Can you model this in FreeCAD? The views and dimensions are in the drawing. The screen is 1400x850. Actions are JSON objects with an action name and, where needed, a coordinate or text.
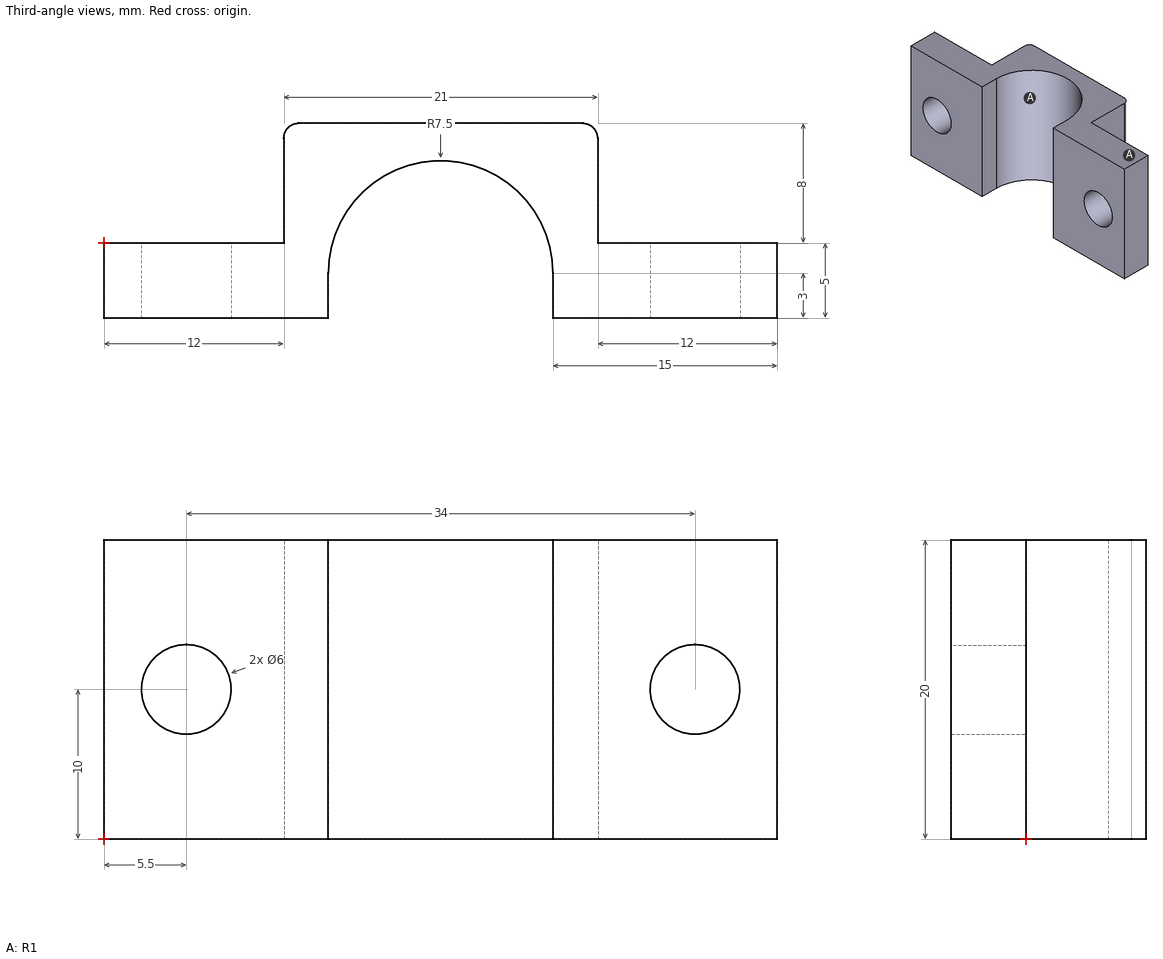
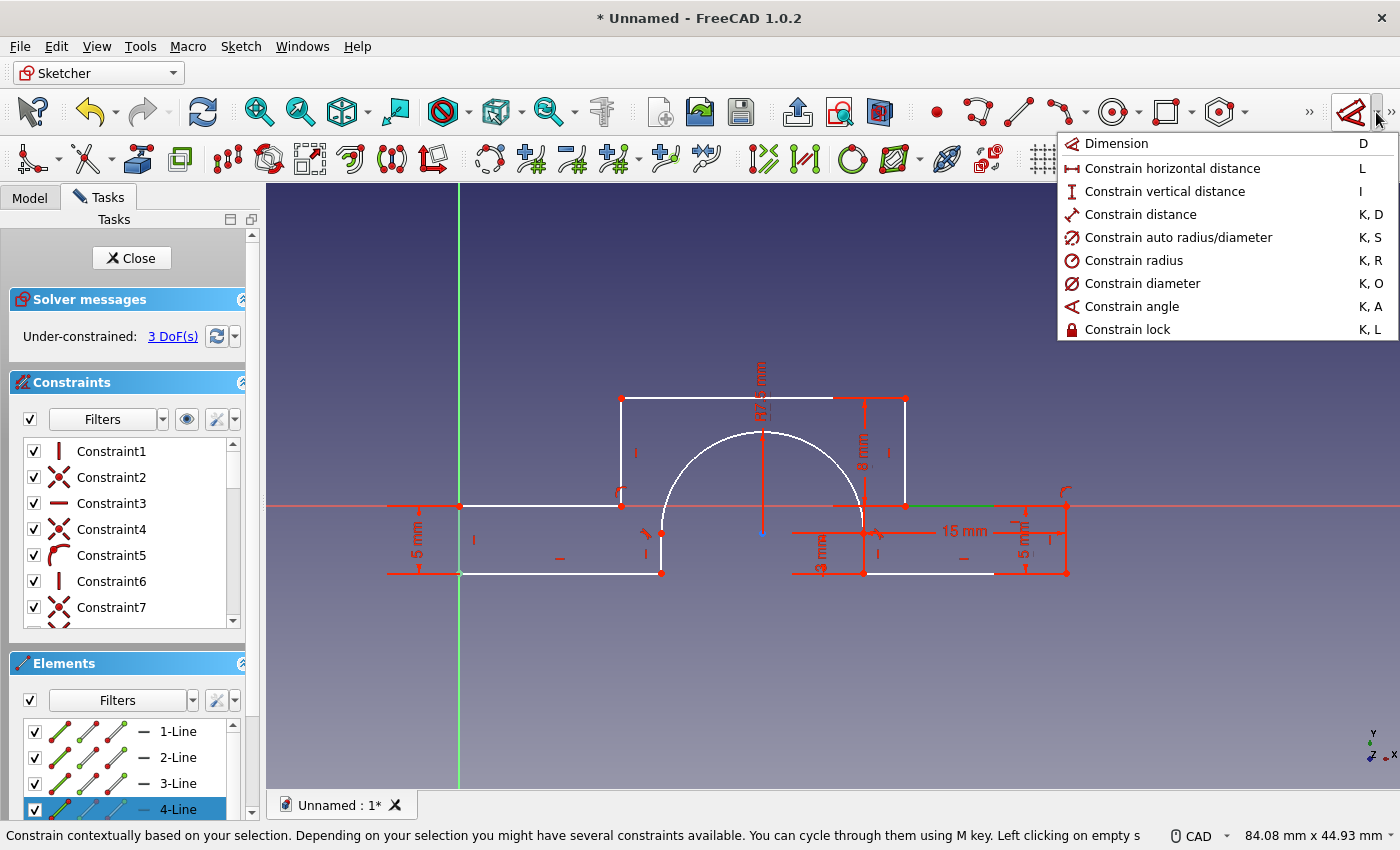
{"action": "left_click", "coordinate": [1228, 168]}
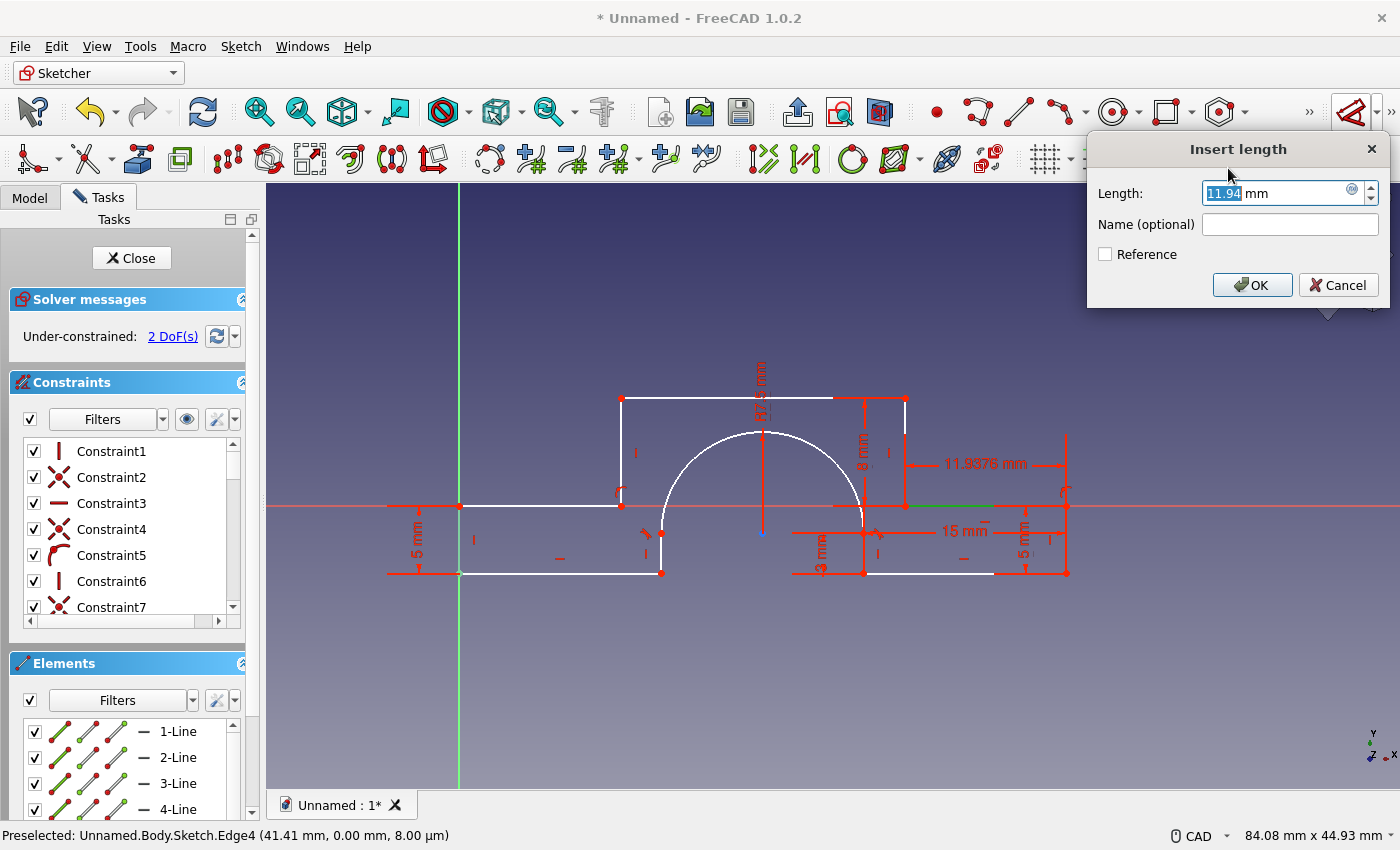
{"action": "type", "text": "12"}
{"action": "key", "text": "Return"}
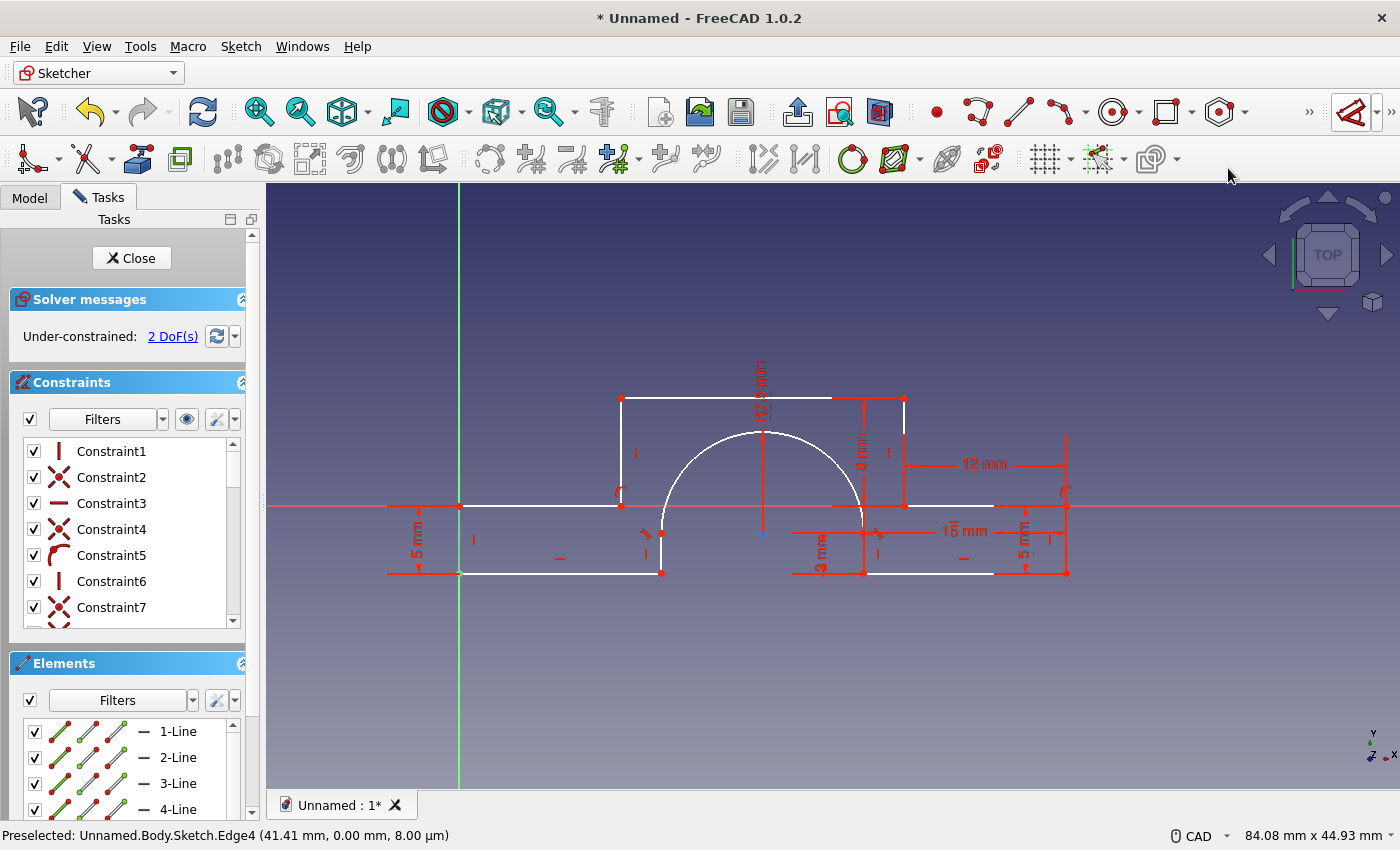
{"action": "left_click", "coordinate": [819, 398]}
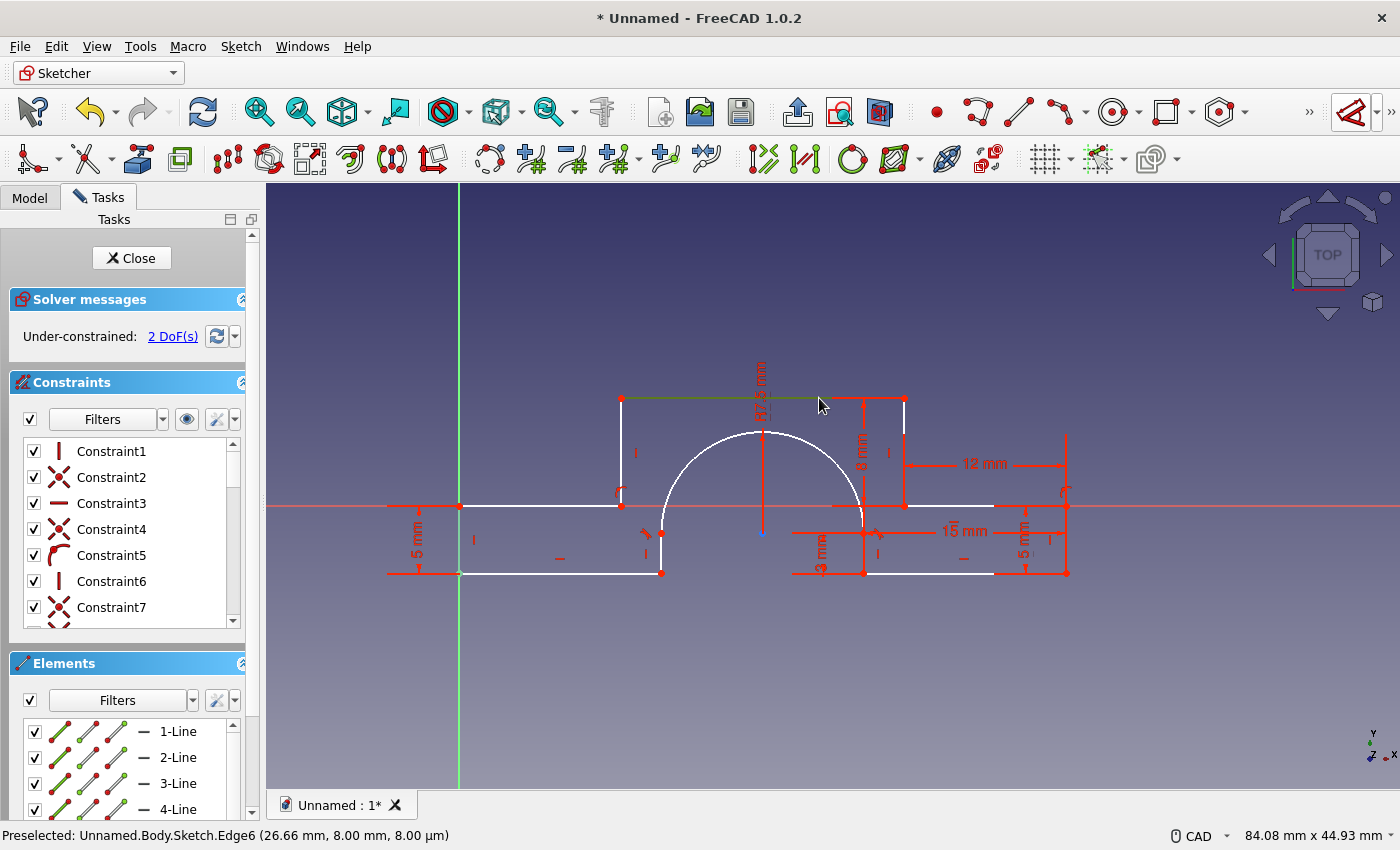
{"action": "key", "text": "l"}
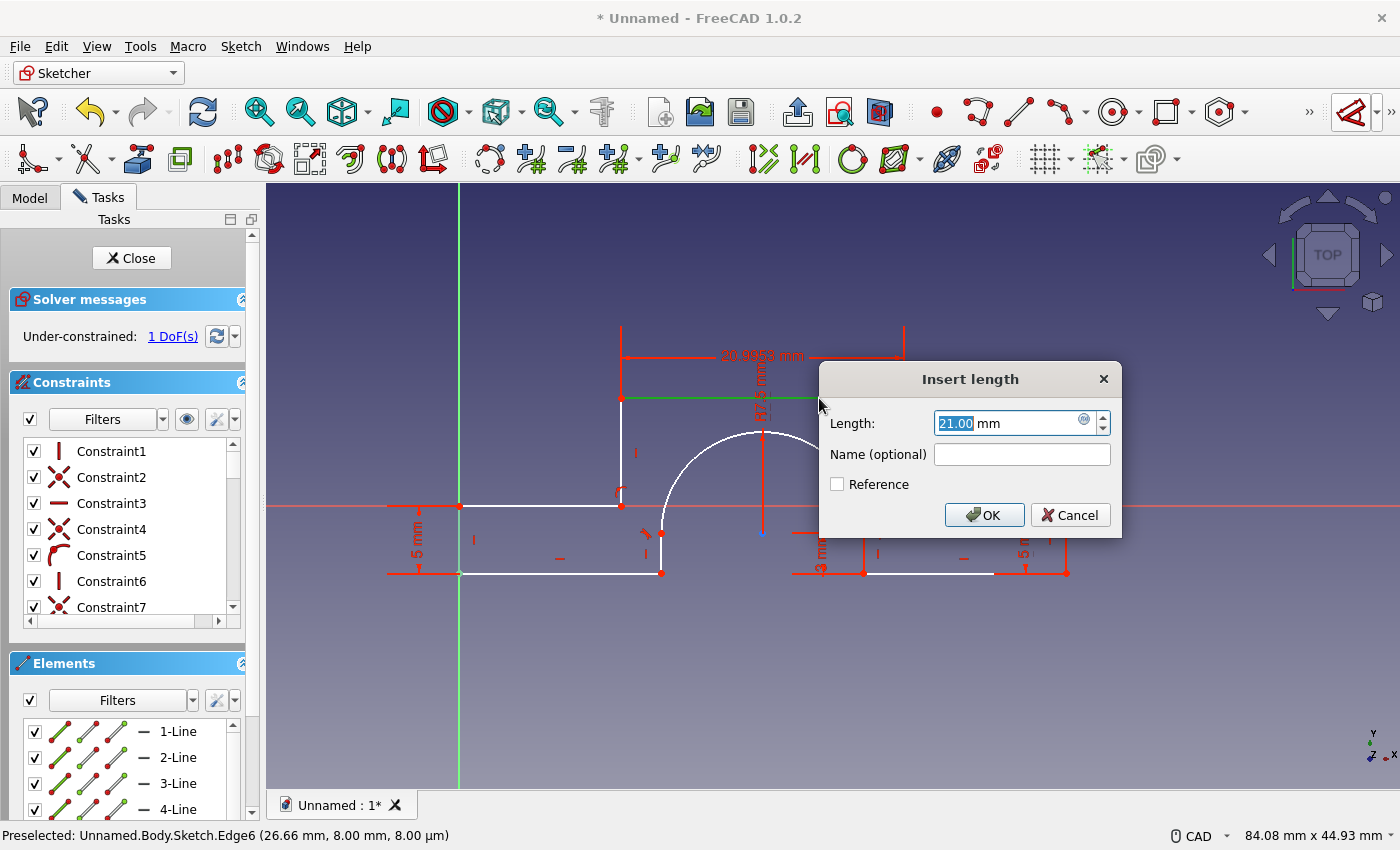
{"action": "type", "text": "21"}
{"action": "key", "text": "Return"}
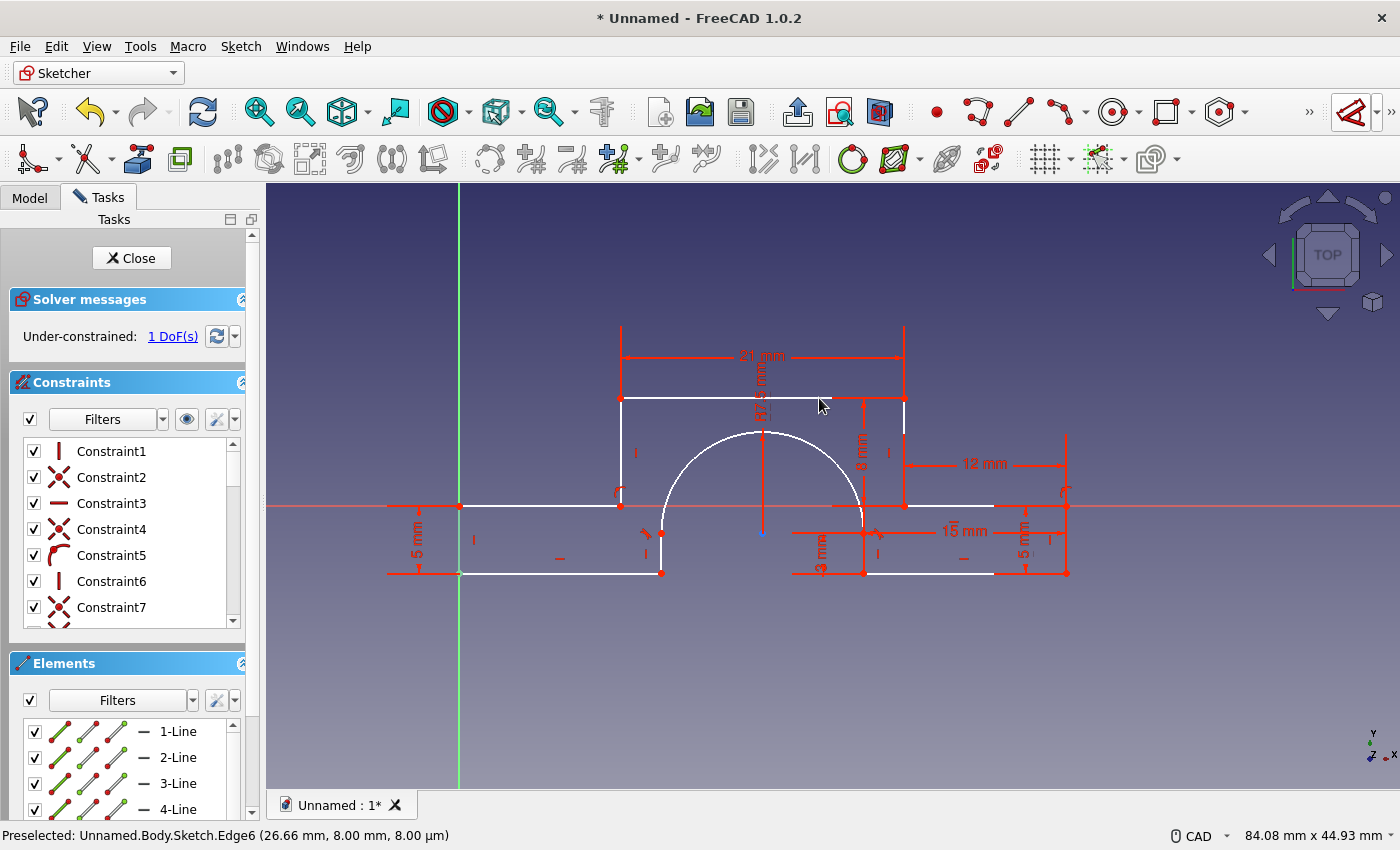
{"action": "left_click", "coordinate": [573, 506]}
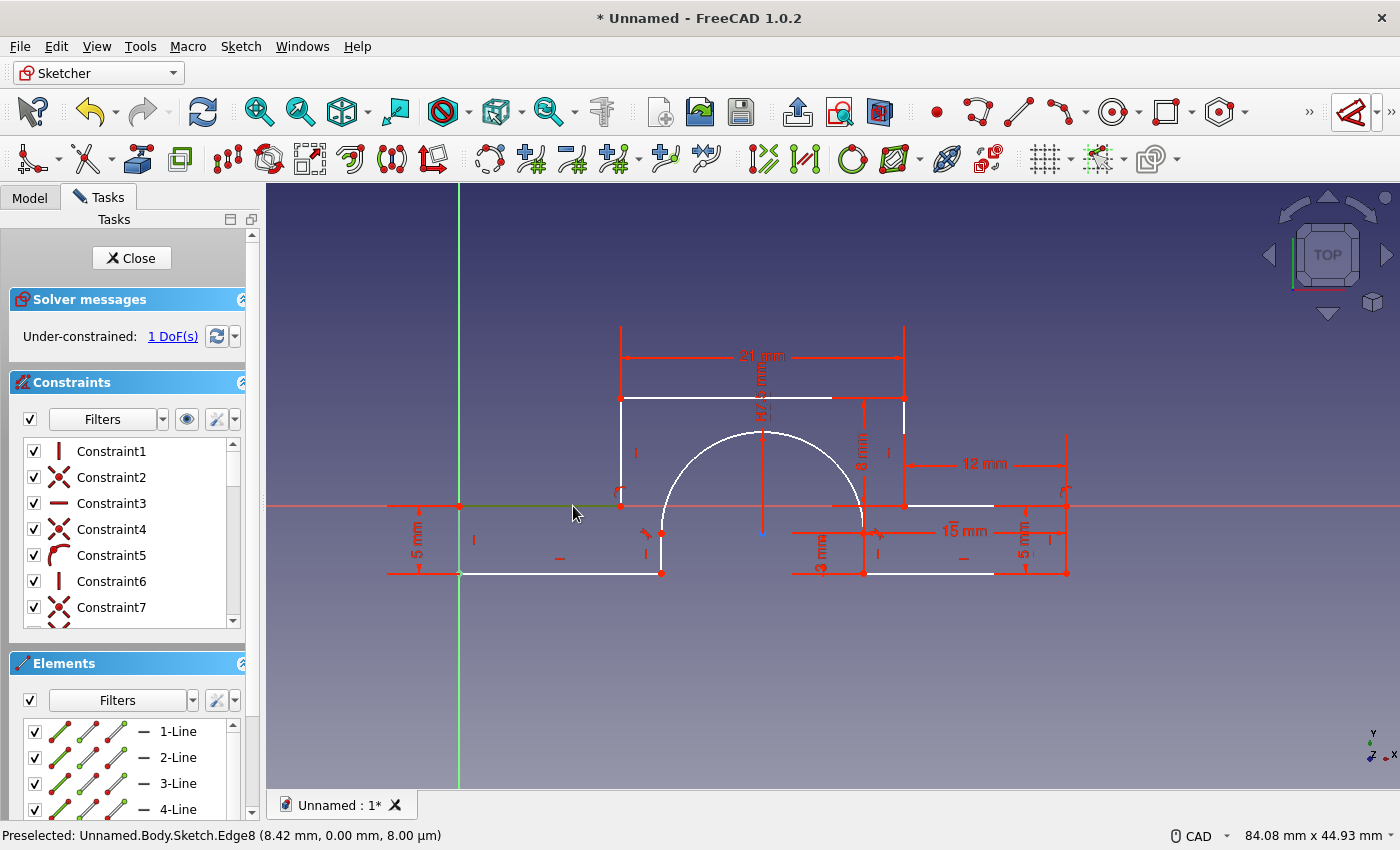
{"action": "left_click", "coordinate": [1376, 112]}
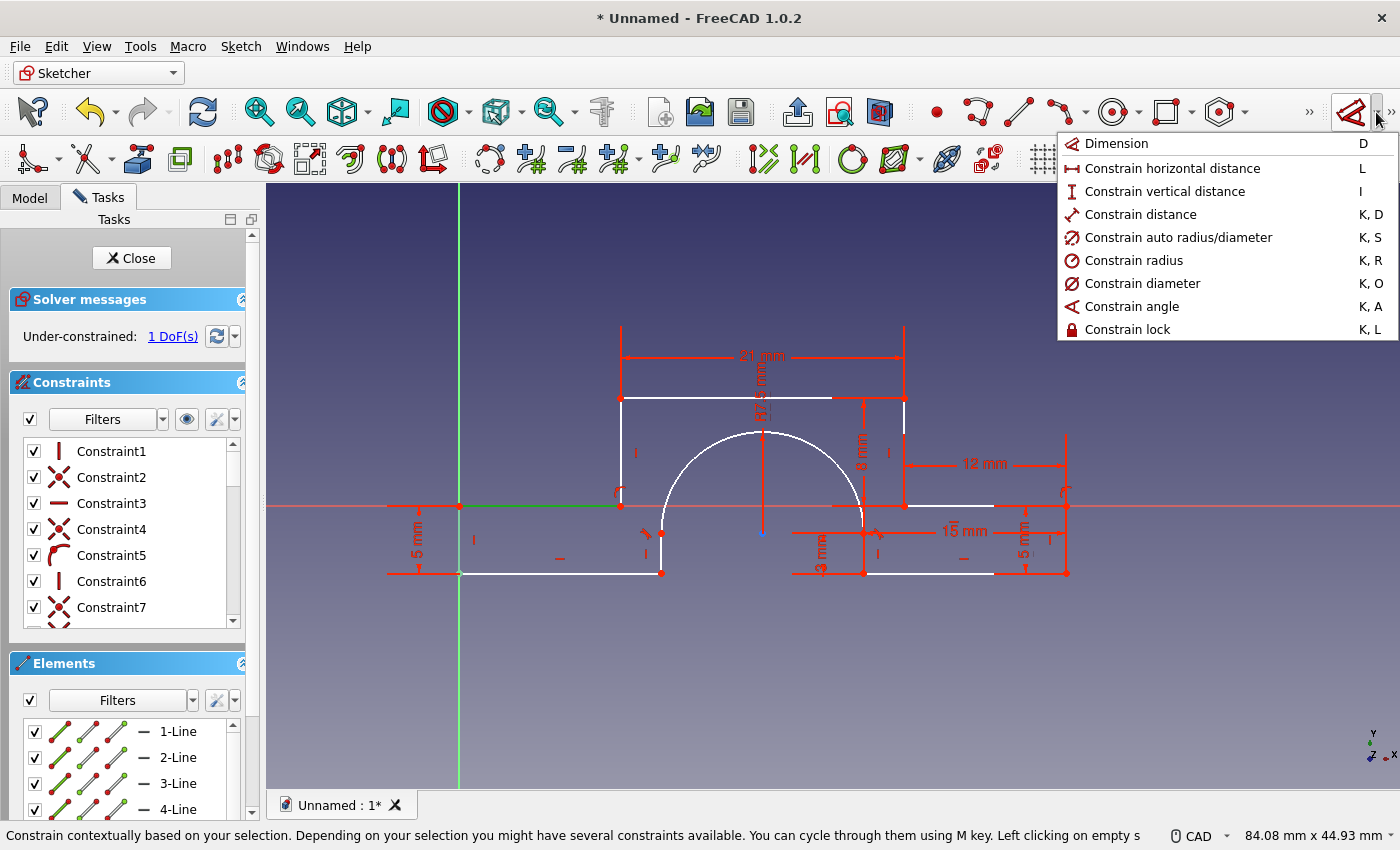
{"action": "left_click", "coordinate": [1228, 168]}